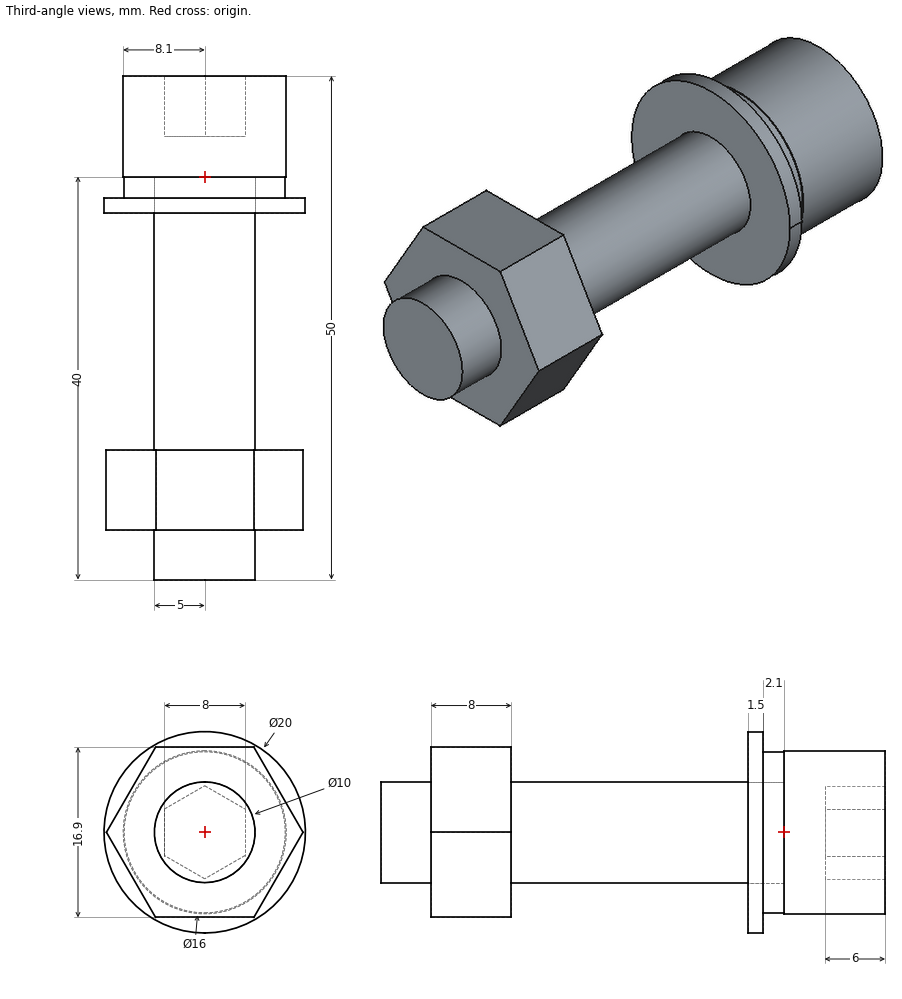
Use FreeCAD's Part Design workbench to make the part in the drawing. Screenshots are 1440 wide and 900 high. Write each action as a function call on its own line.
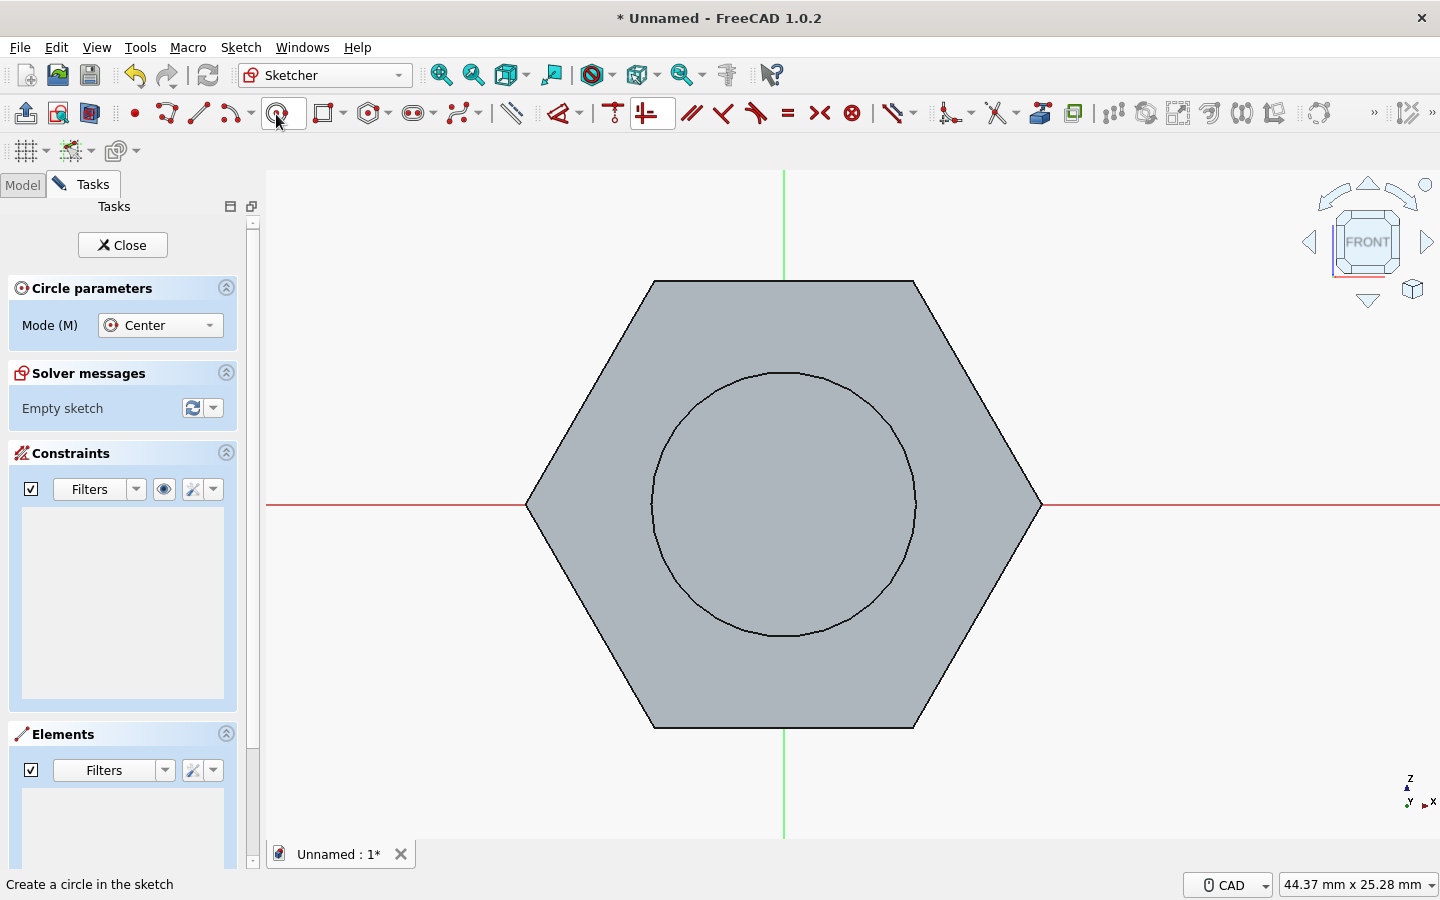
click(784, 504)
move(933, 355)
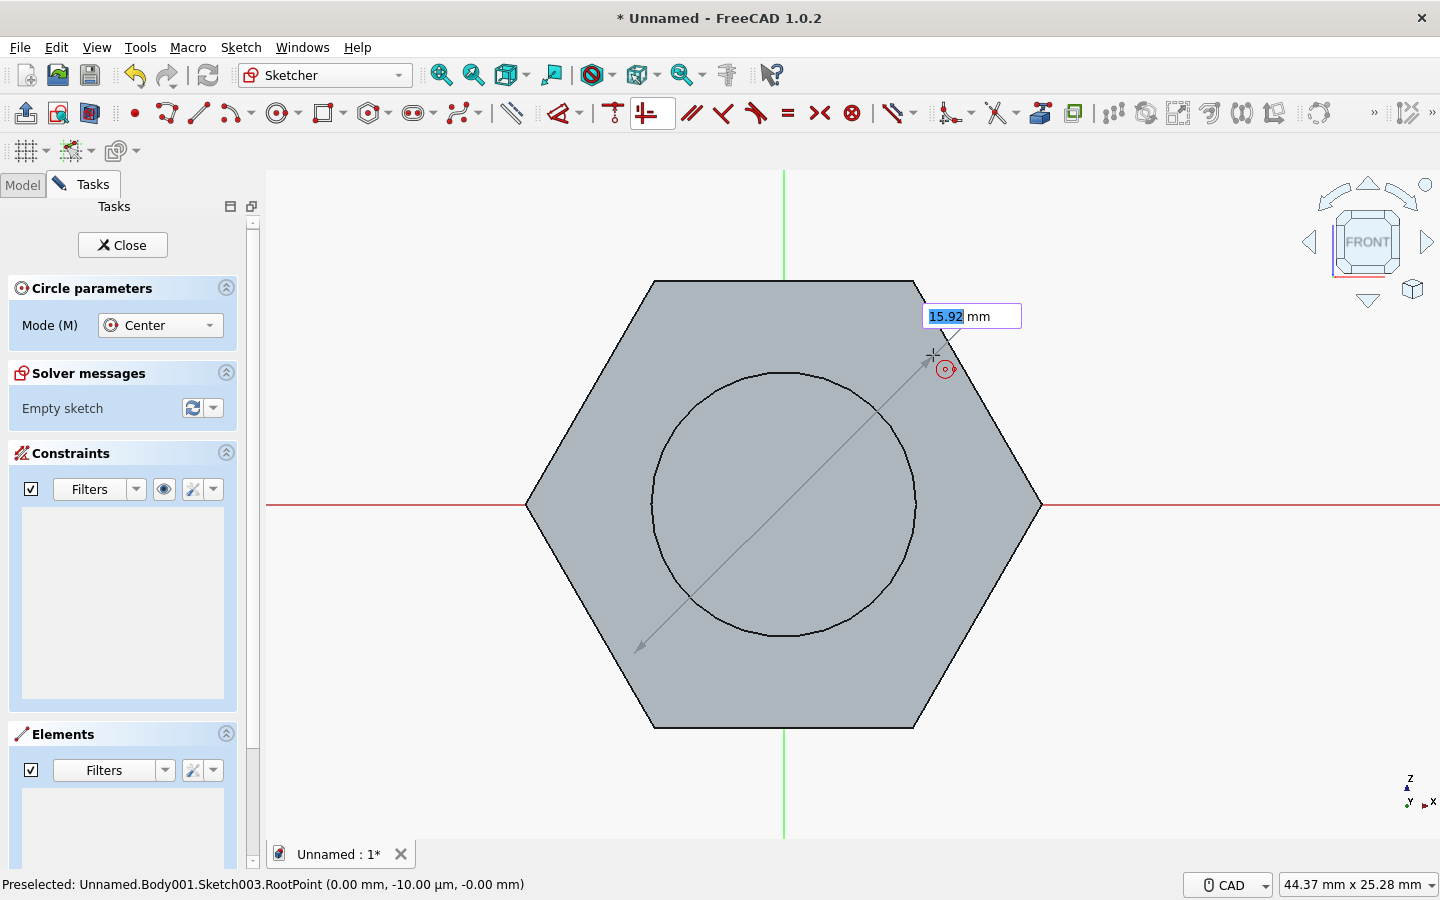
text(16)
key(Return)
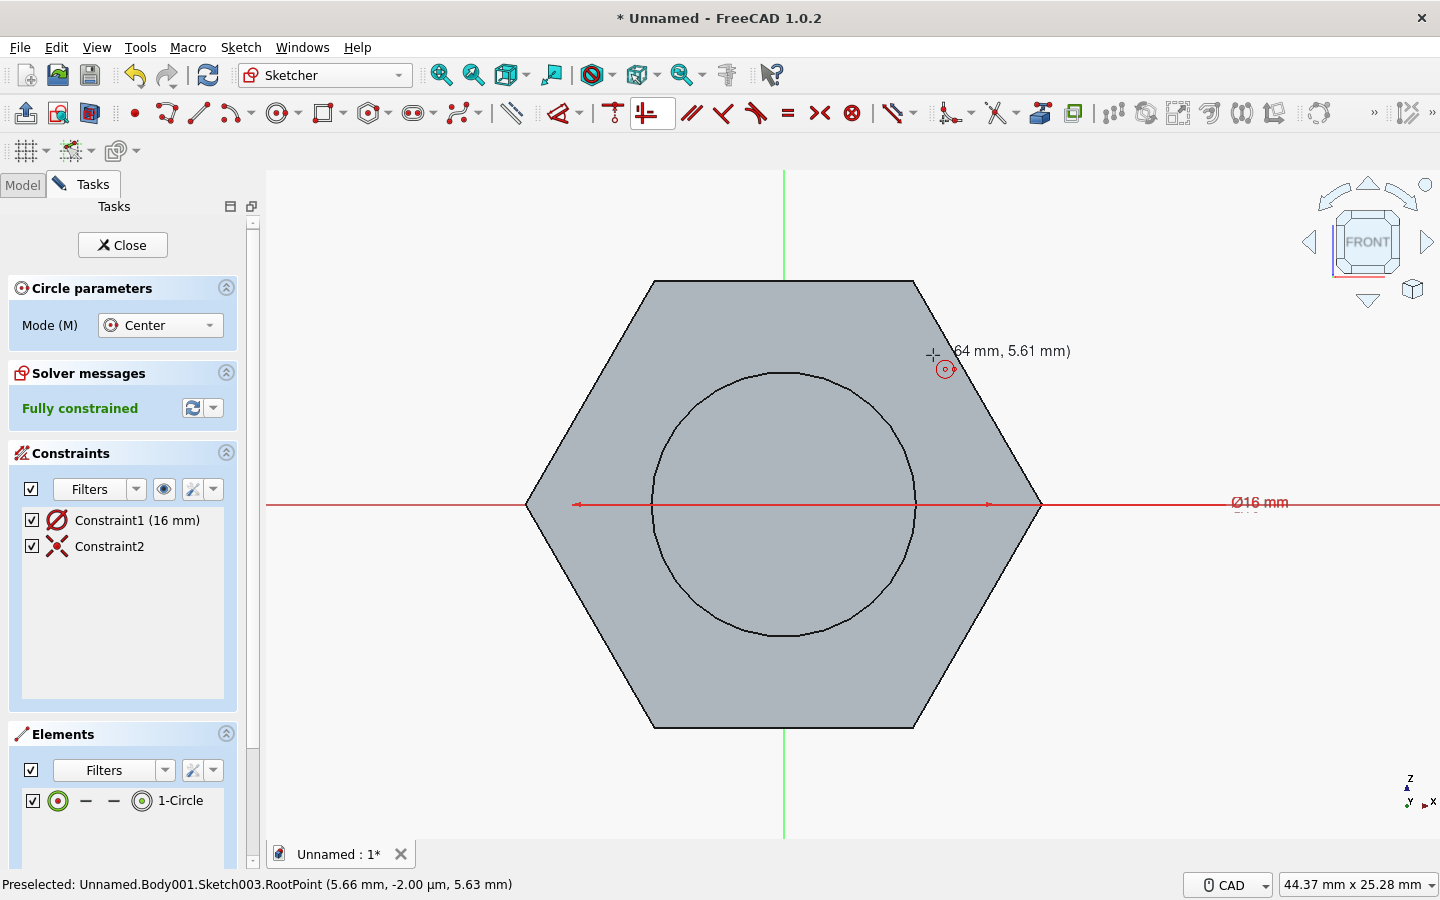
click(784, 504)
move(877, 411)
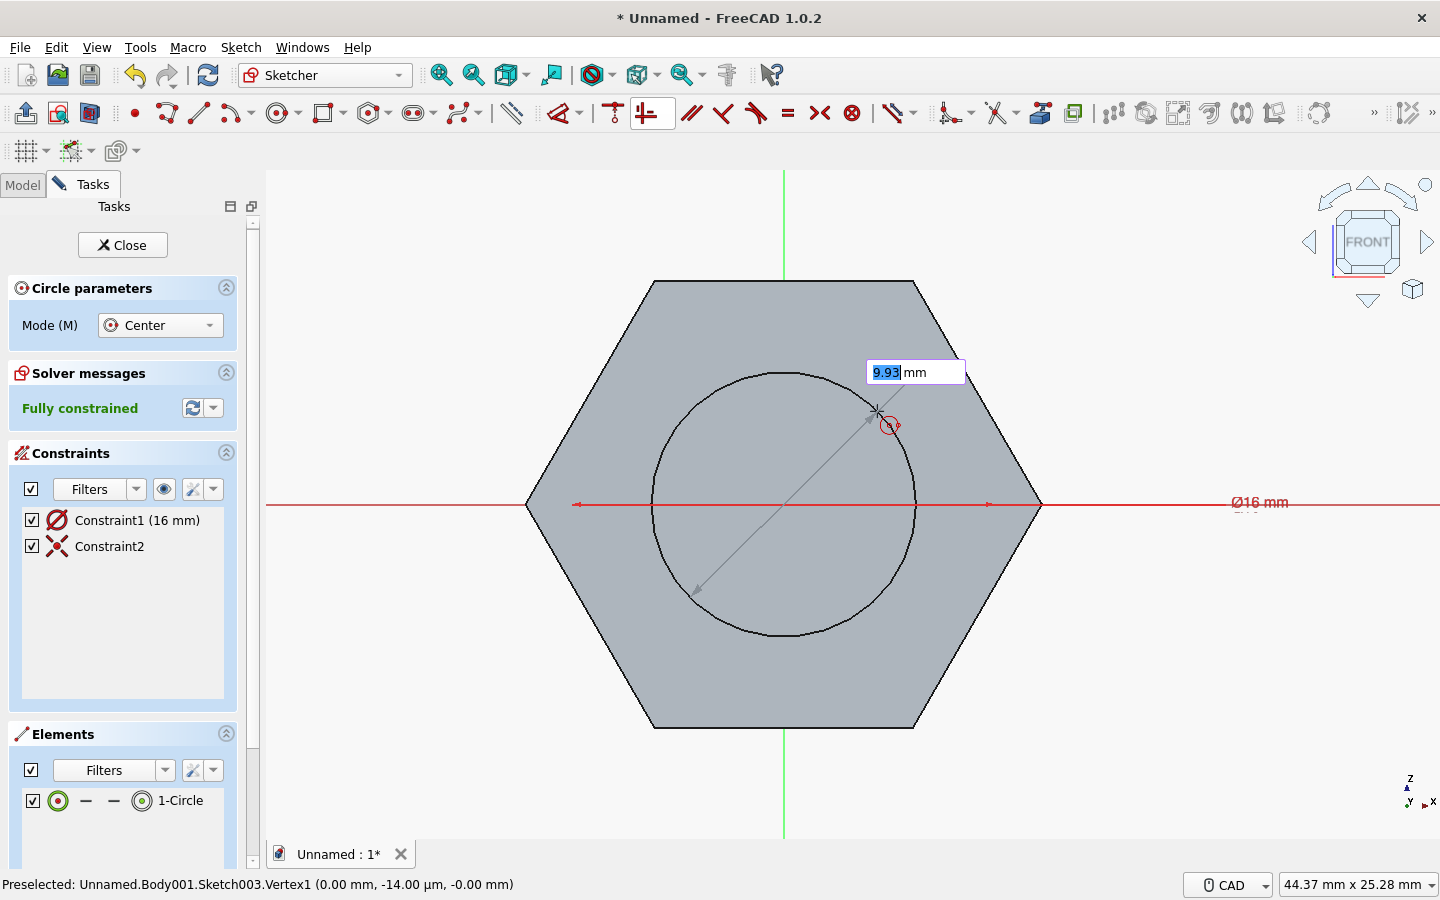
text(10)
key(Return)
key(Escape)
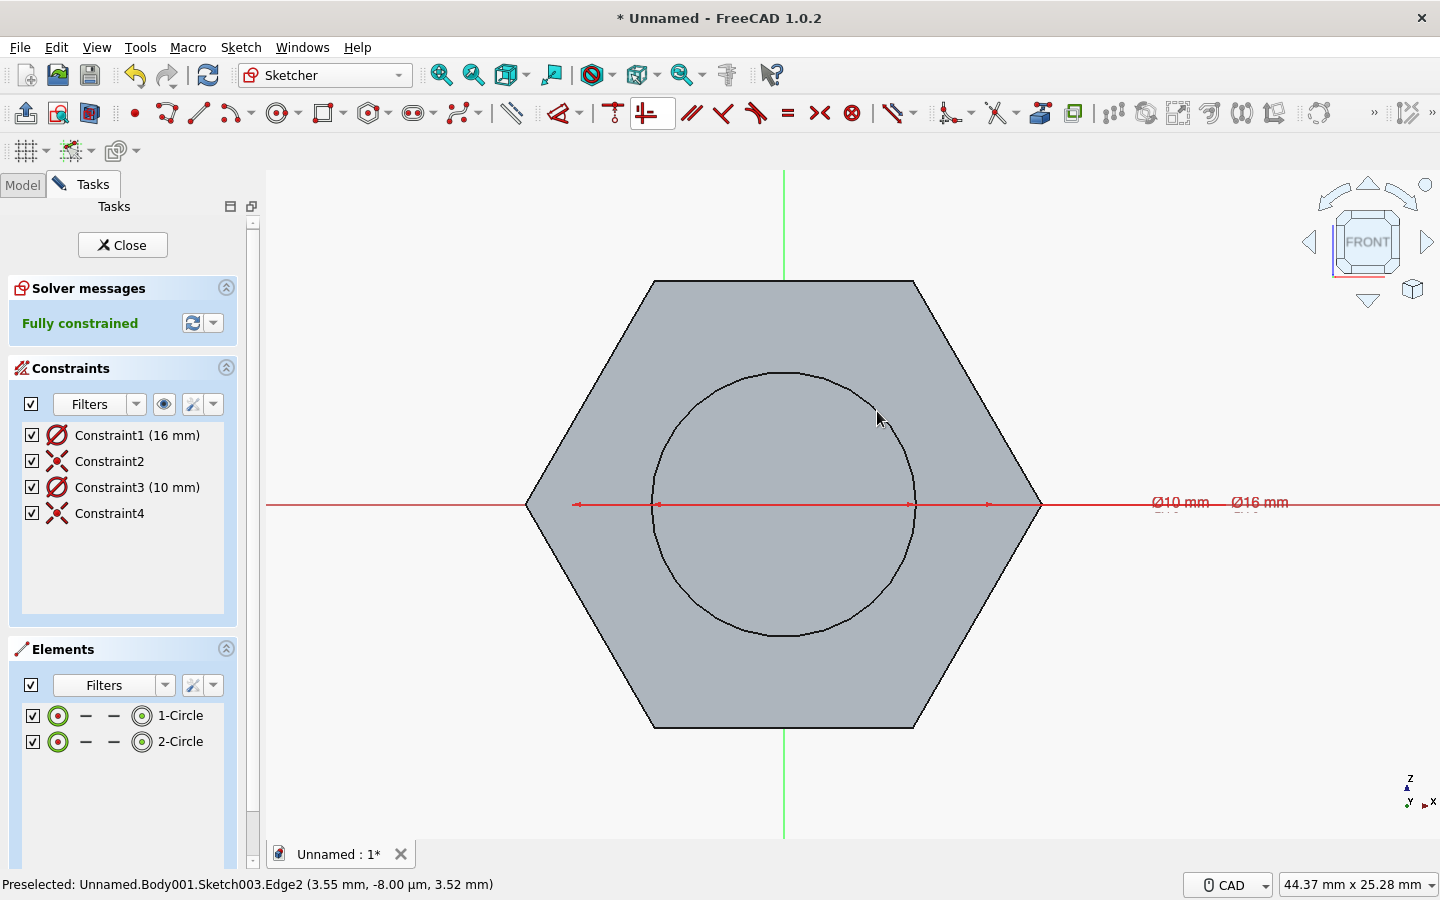
click(123, 245)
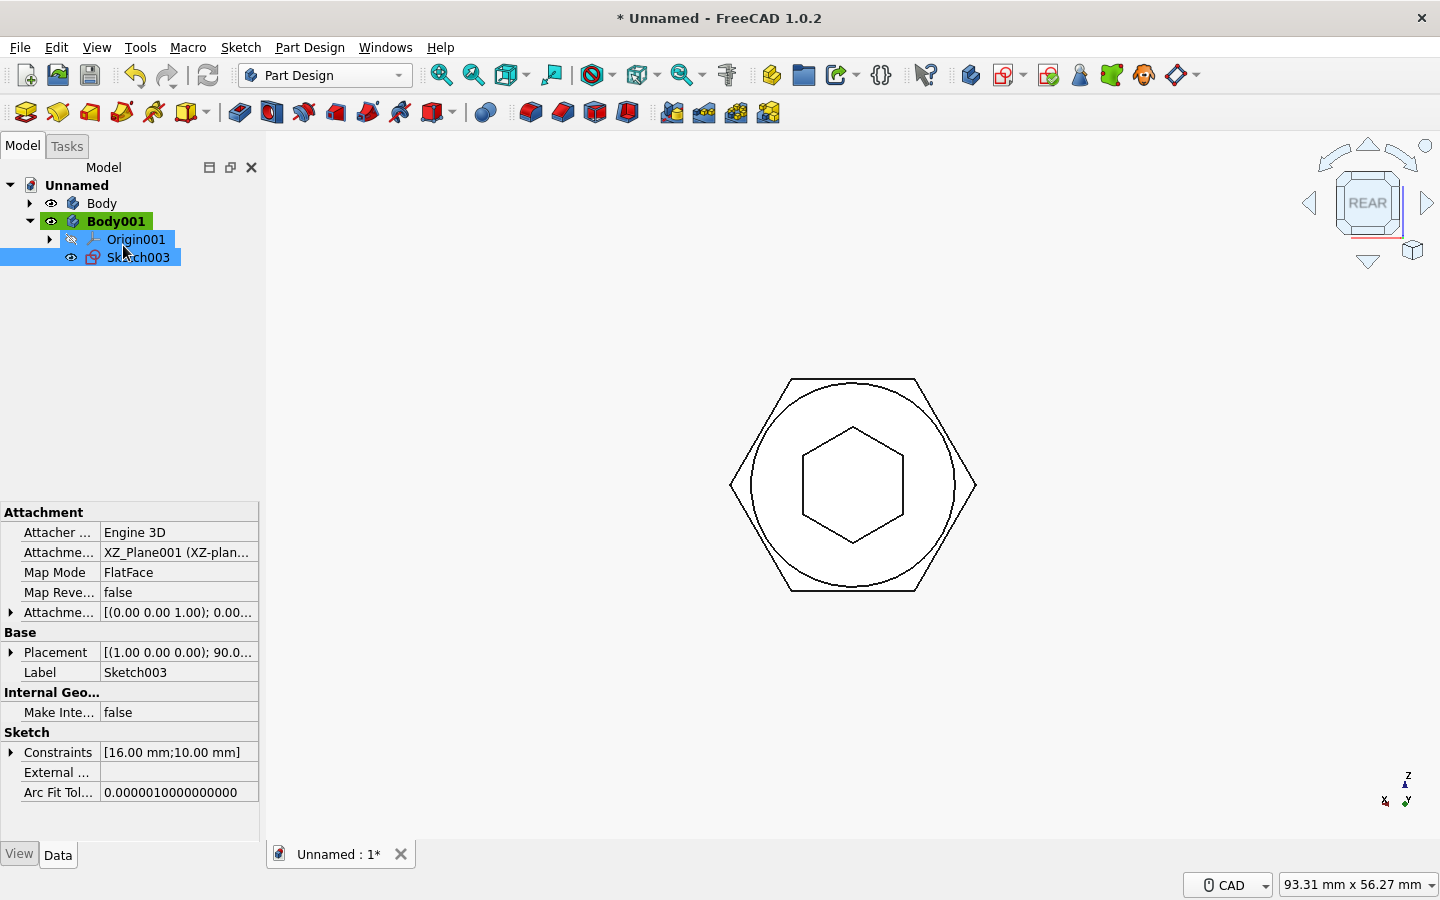
click(26, 112)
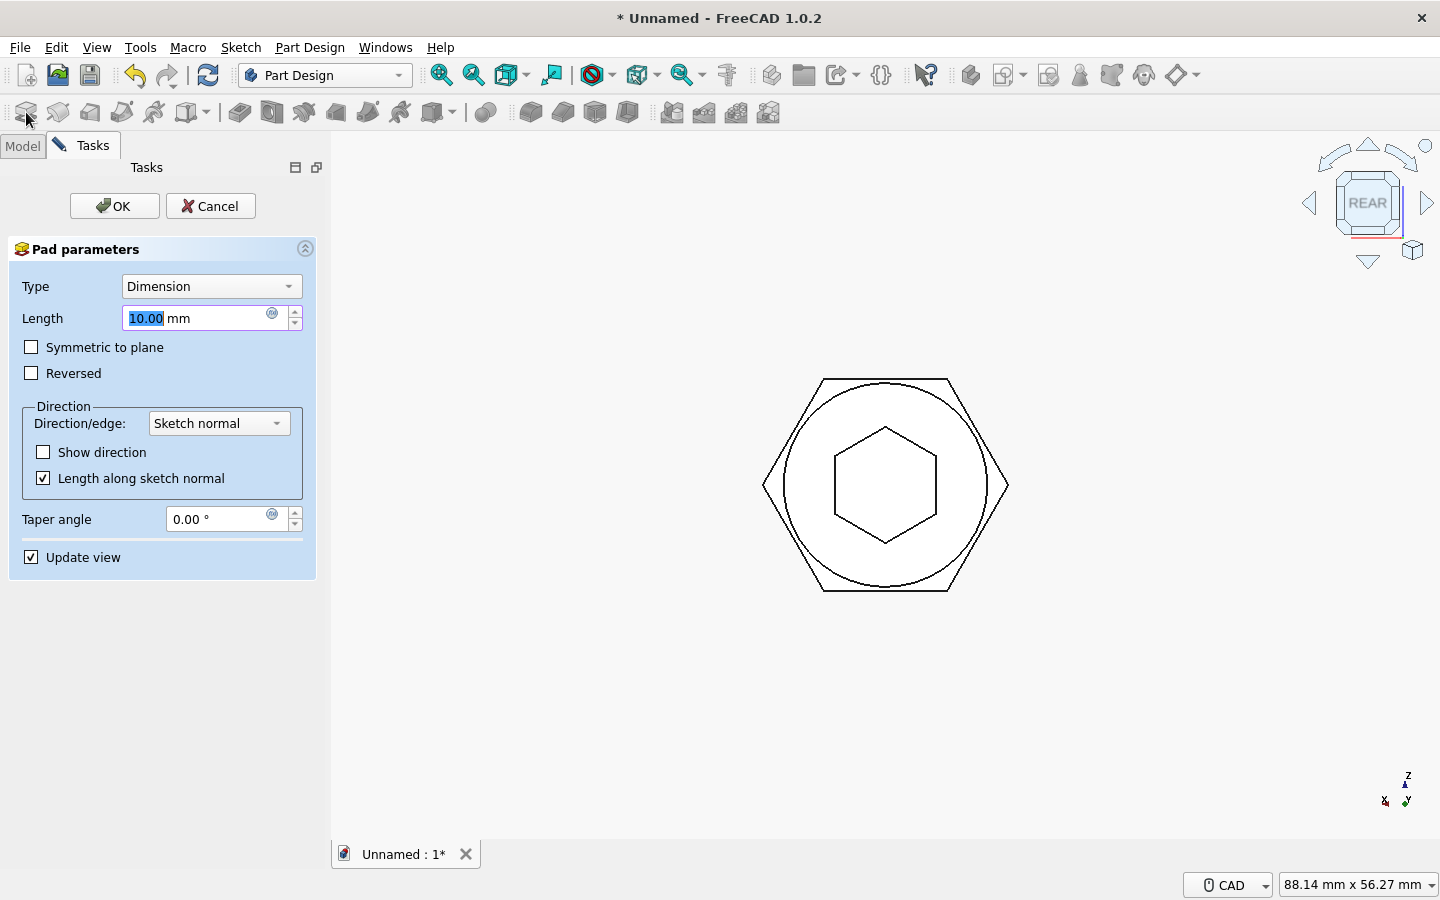
text(2.1)
key(Tab)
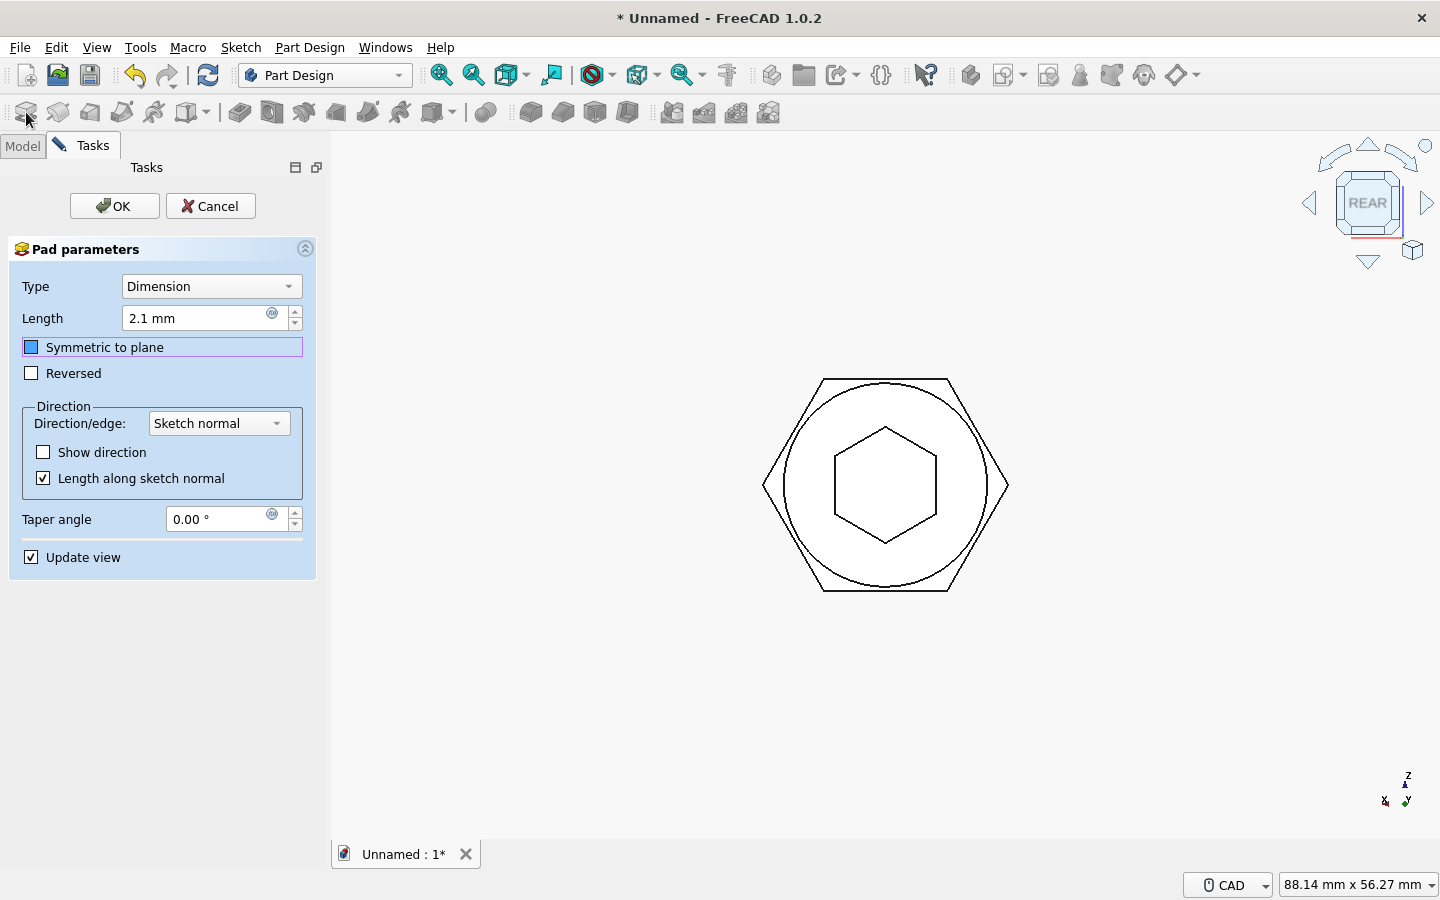
click(115, 206)